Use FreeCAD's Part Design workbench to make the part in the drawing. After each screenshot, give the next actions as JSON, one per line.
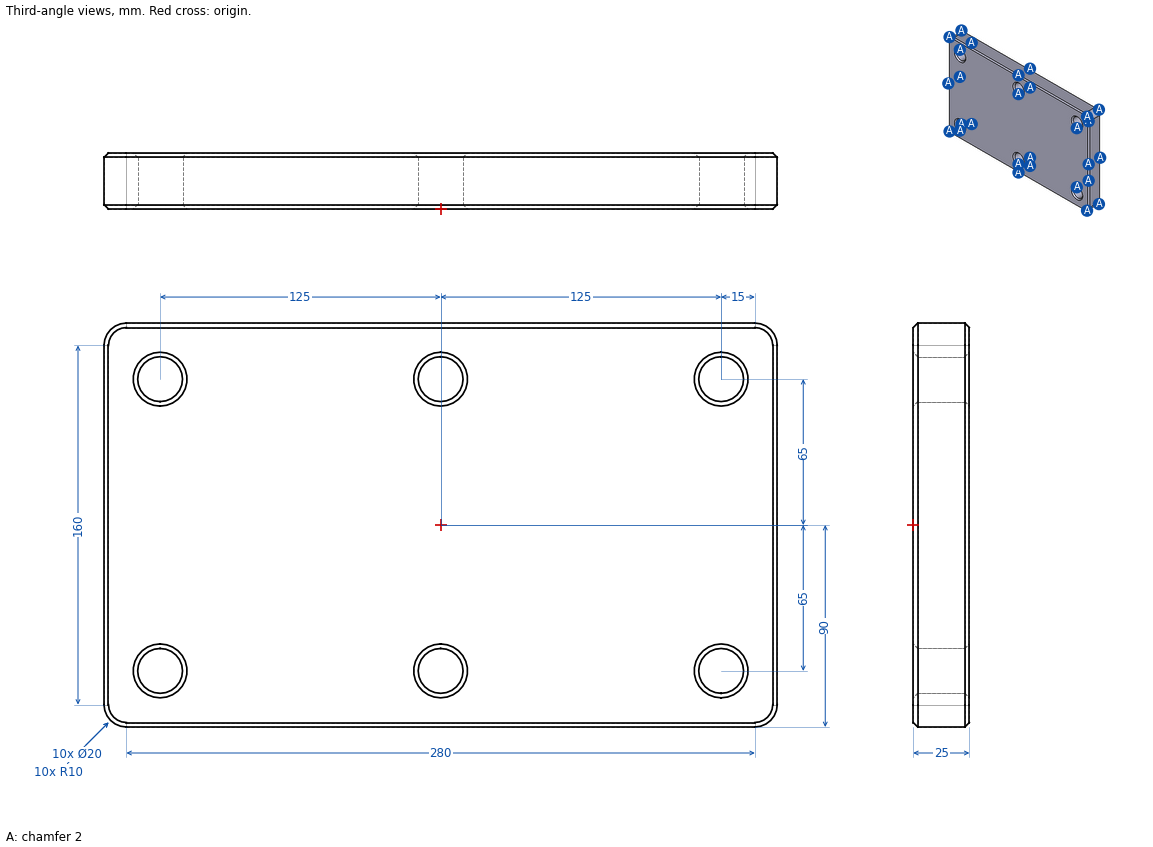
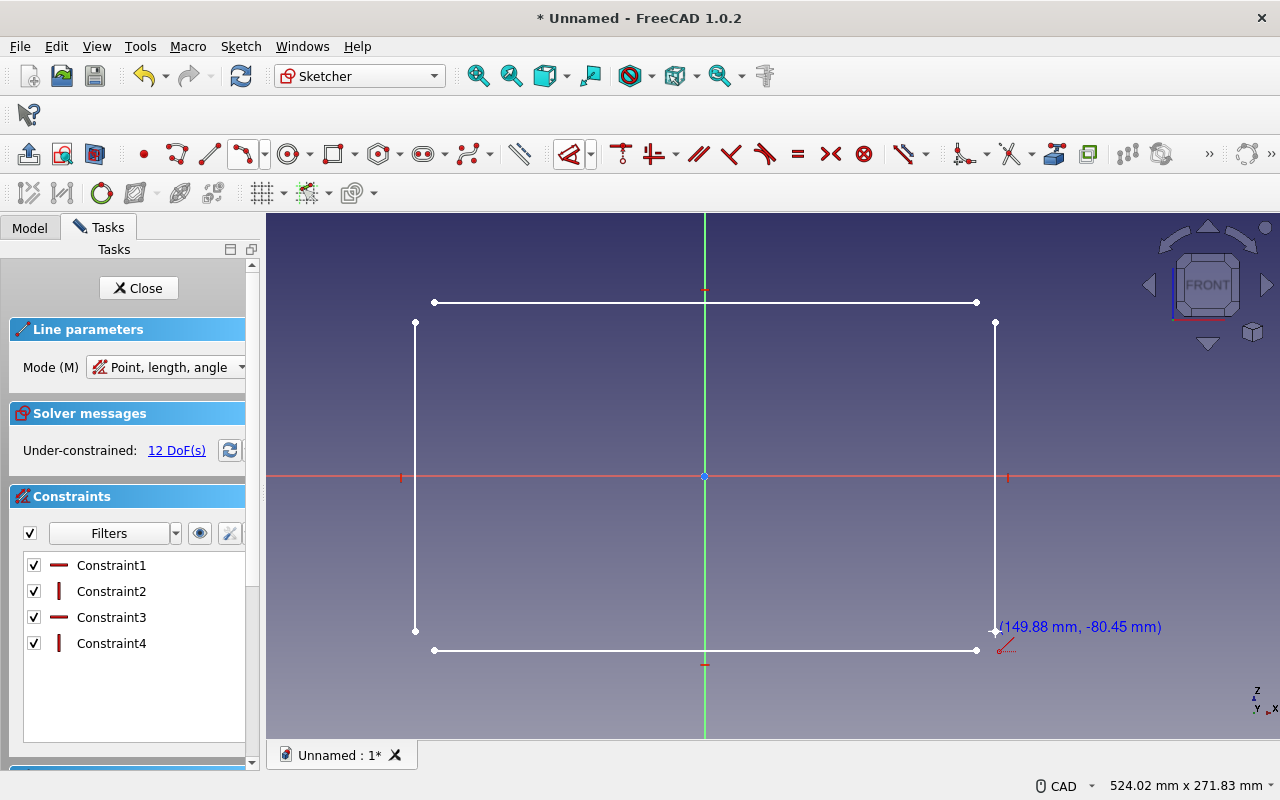
{"action": "left_click", "coordinate": [242, 154]}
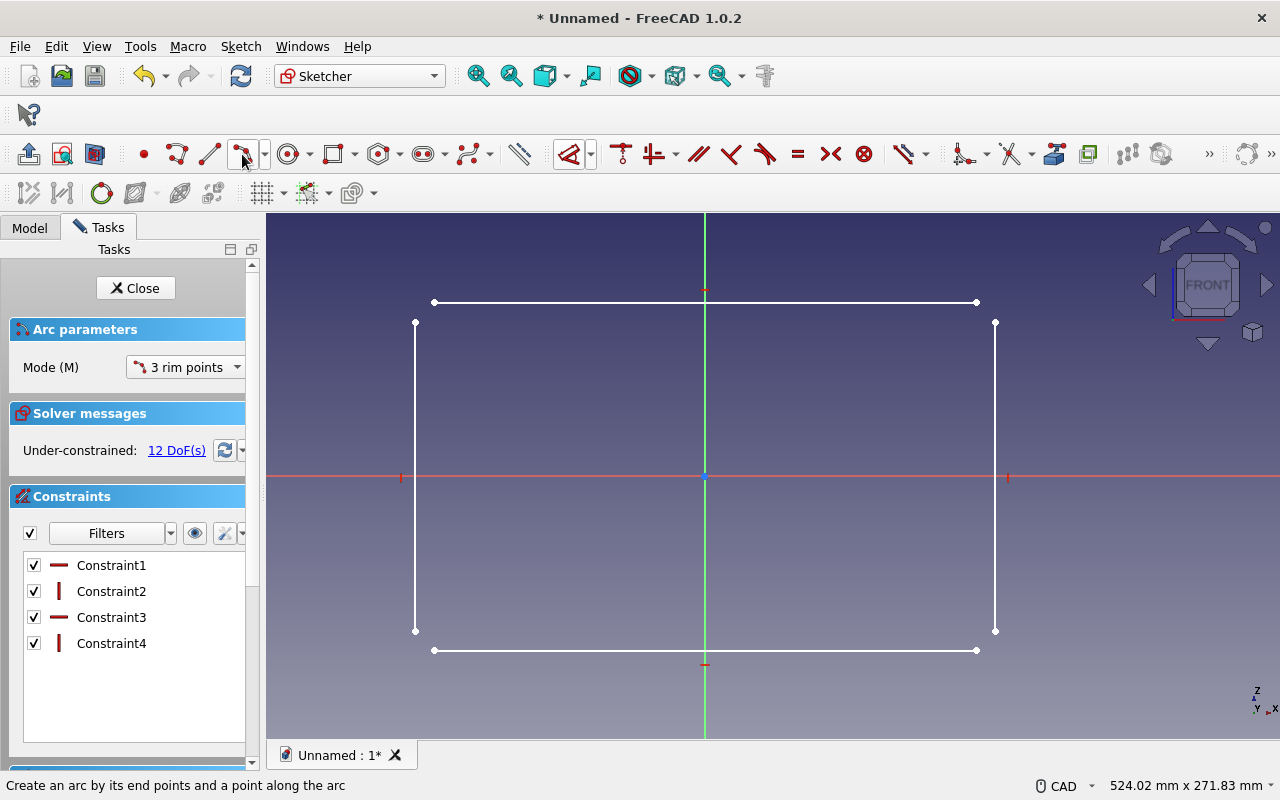
{"action": "left_click", "coordinate": [434, 651]}
{"action": "left_click", "coordinate": [415, 632]}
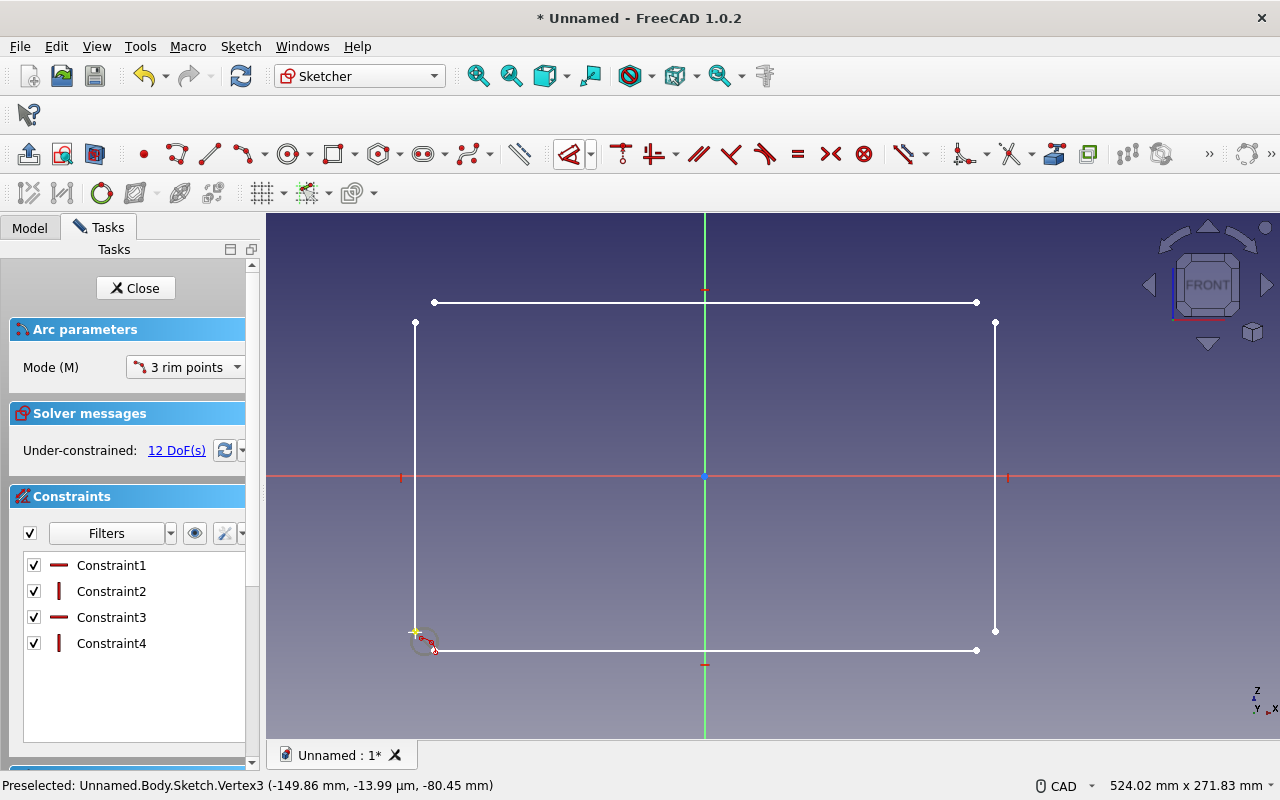
{"action": "scroll", "coordinate": [420, 645], "scroll_direction": "up", "scroll_amount": 6}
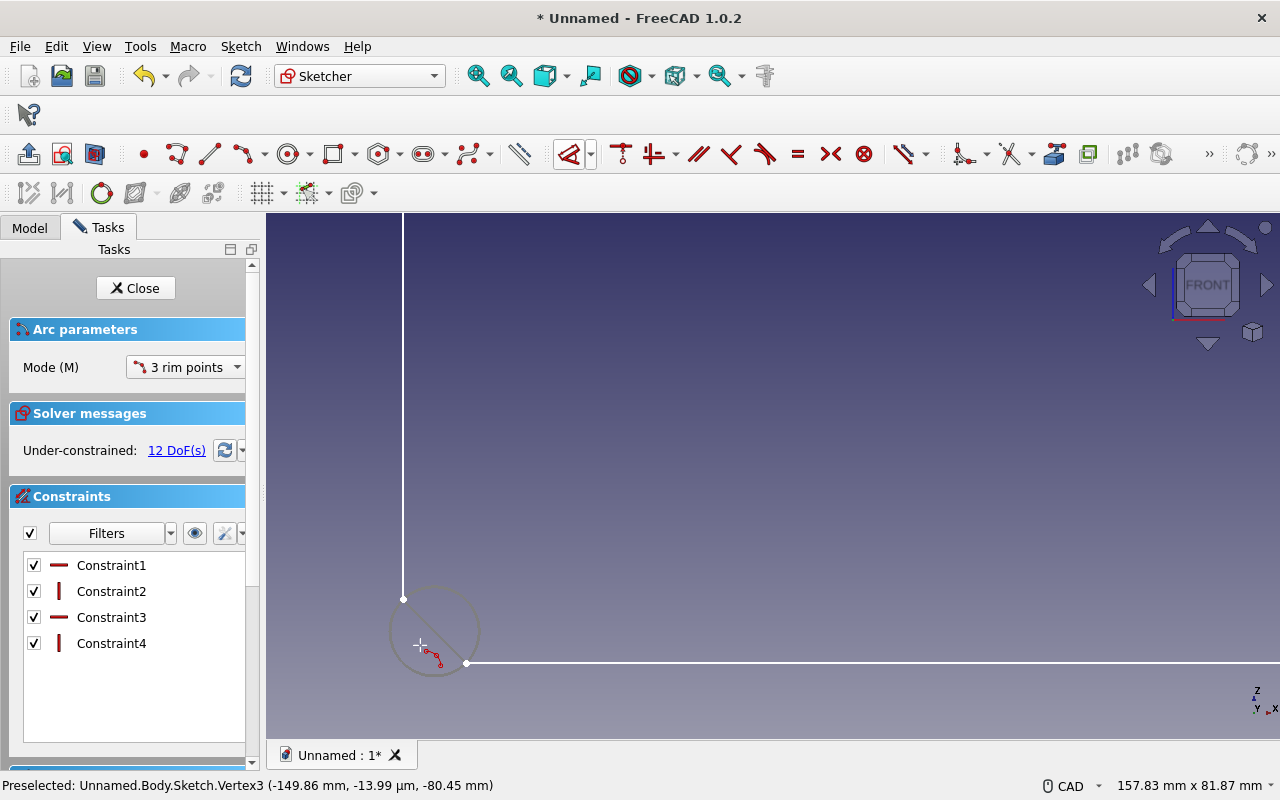
{"action": "left_click", "coordinate": [421, 642]}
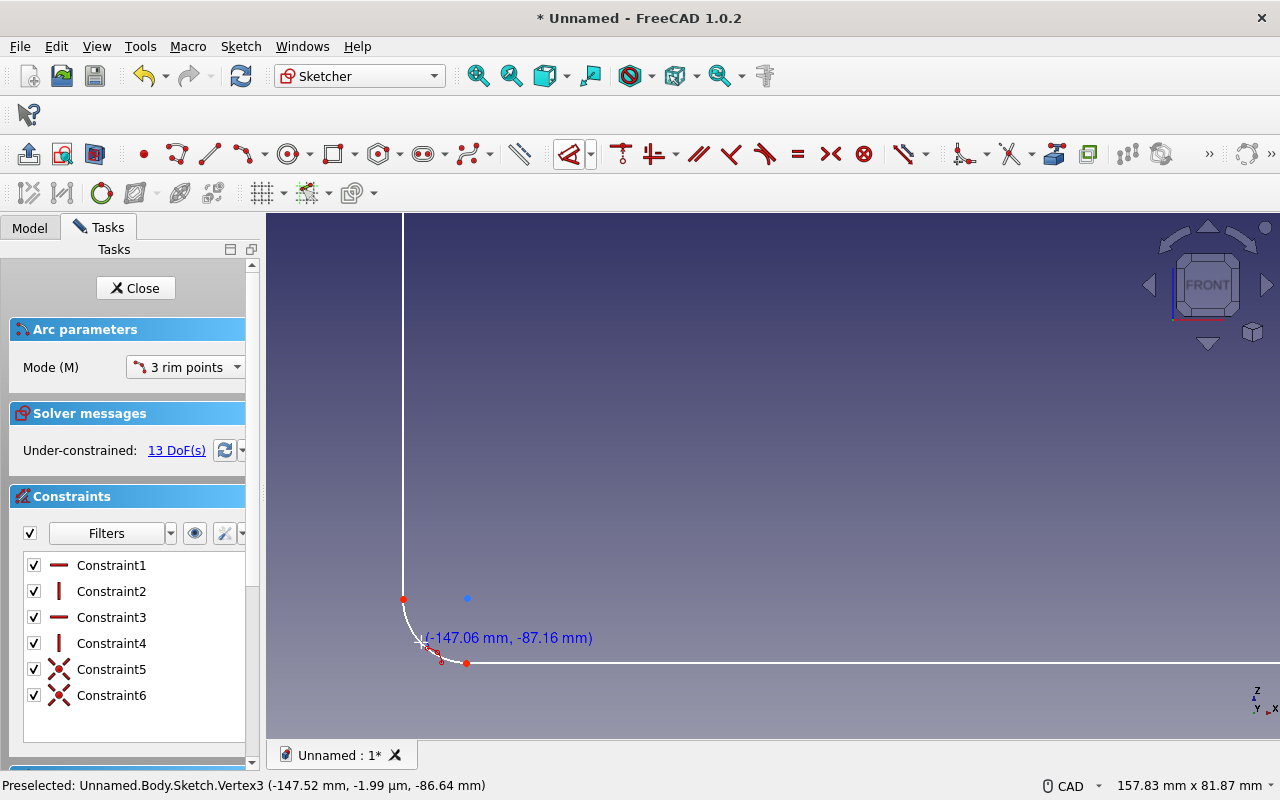
{"action": "scroll", "coordinate": [419, 645], "scroll_direction": "down", "scroll_amount": 6}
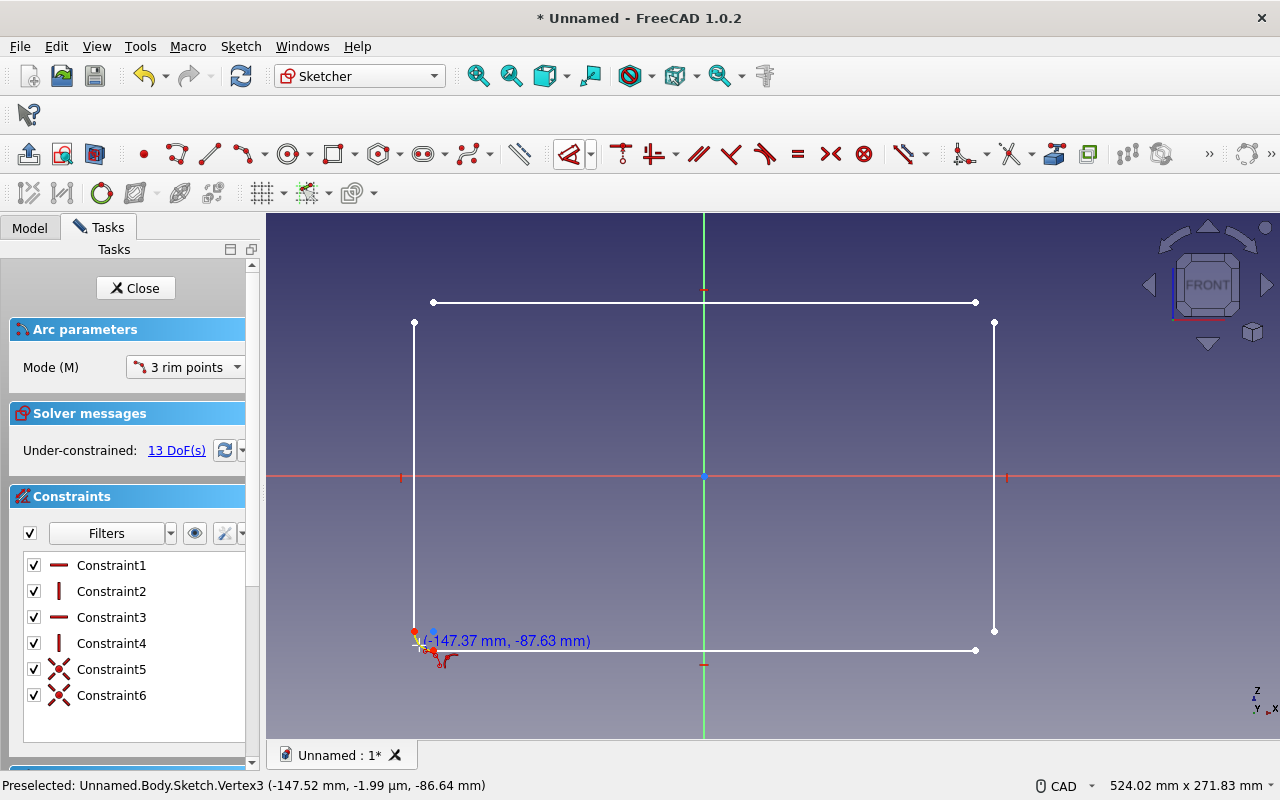
{"action": "left_click", "coordinate": [414, 323]}
{"action": "left_click", "coordinate": [433, 303]}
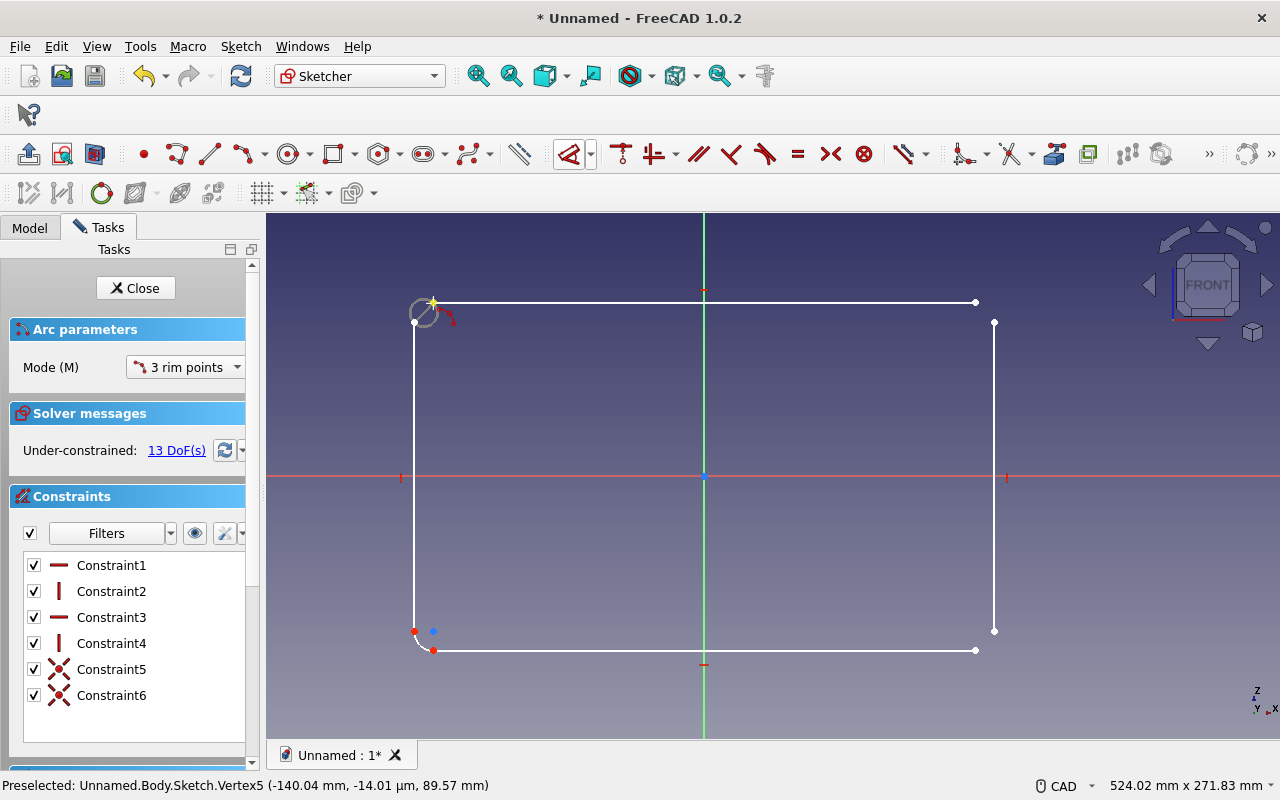
{"action": "scroll", "coordinate": [420, 308], "scroll_direction": "up", "scroll_amount": 6}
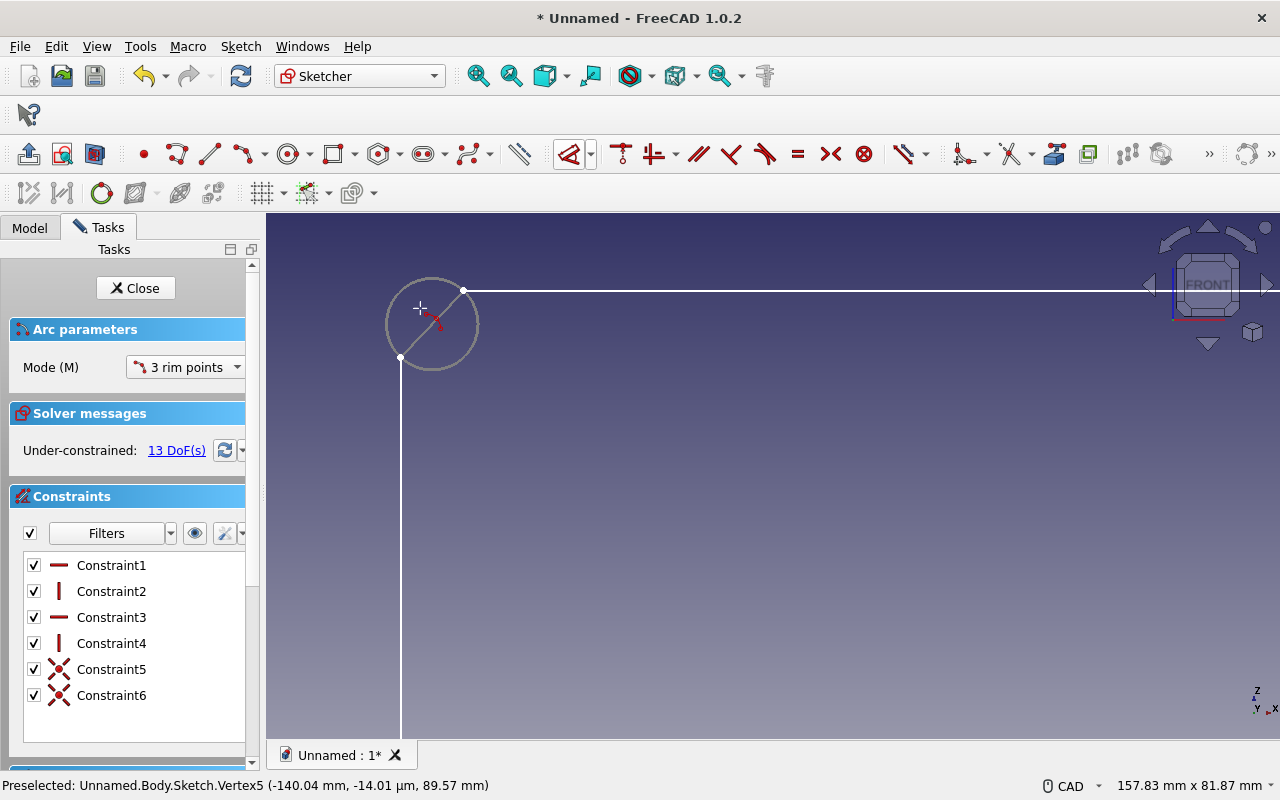
{"action": "left_click", "coordinate": [419, 307]}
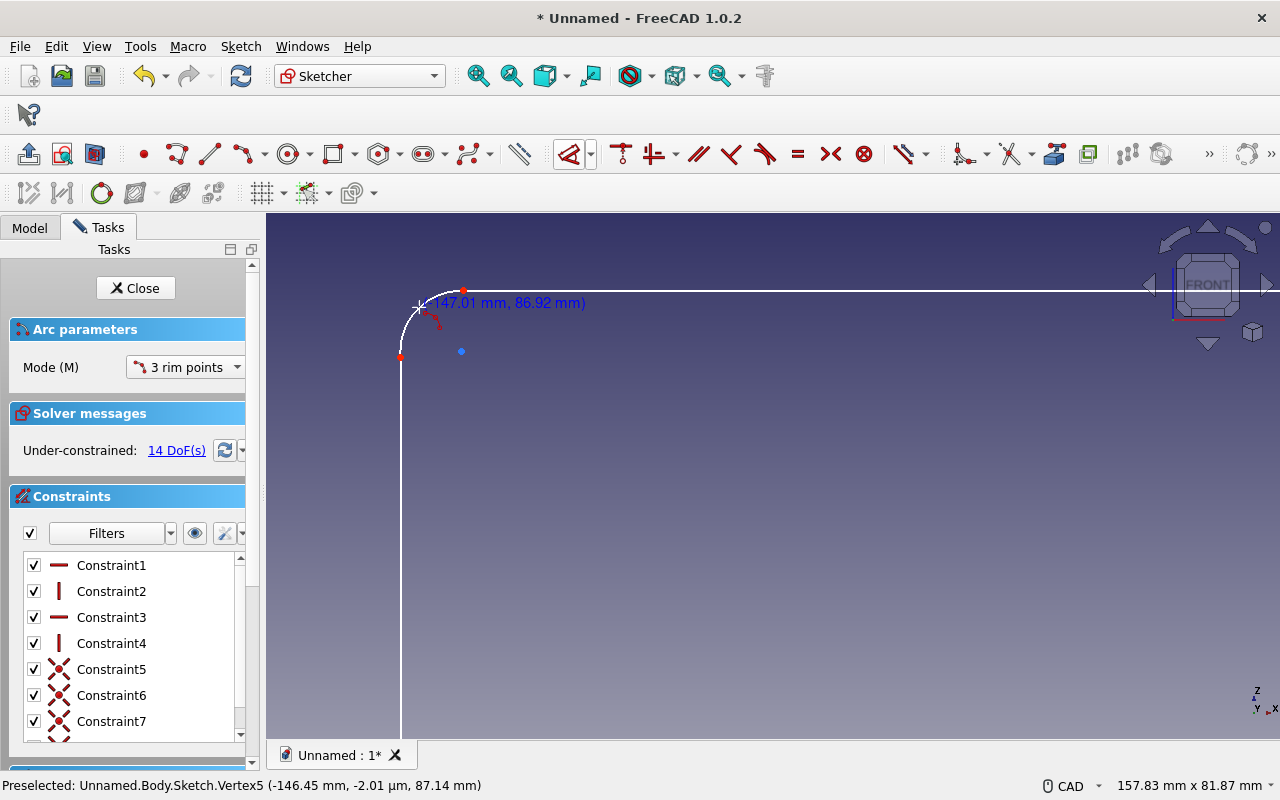
{"action": "scroll", "coordinate": [420, 308], "scroll_direction": "down", "scroll_amount": 6}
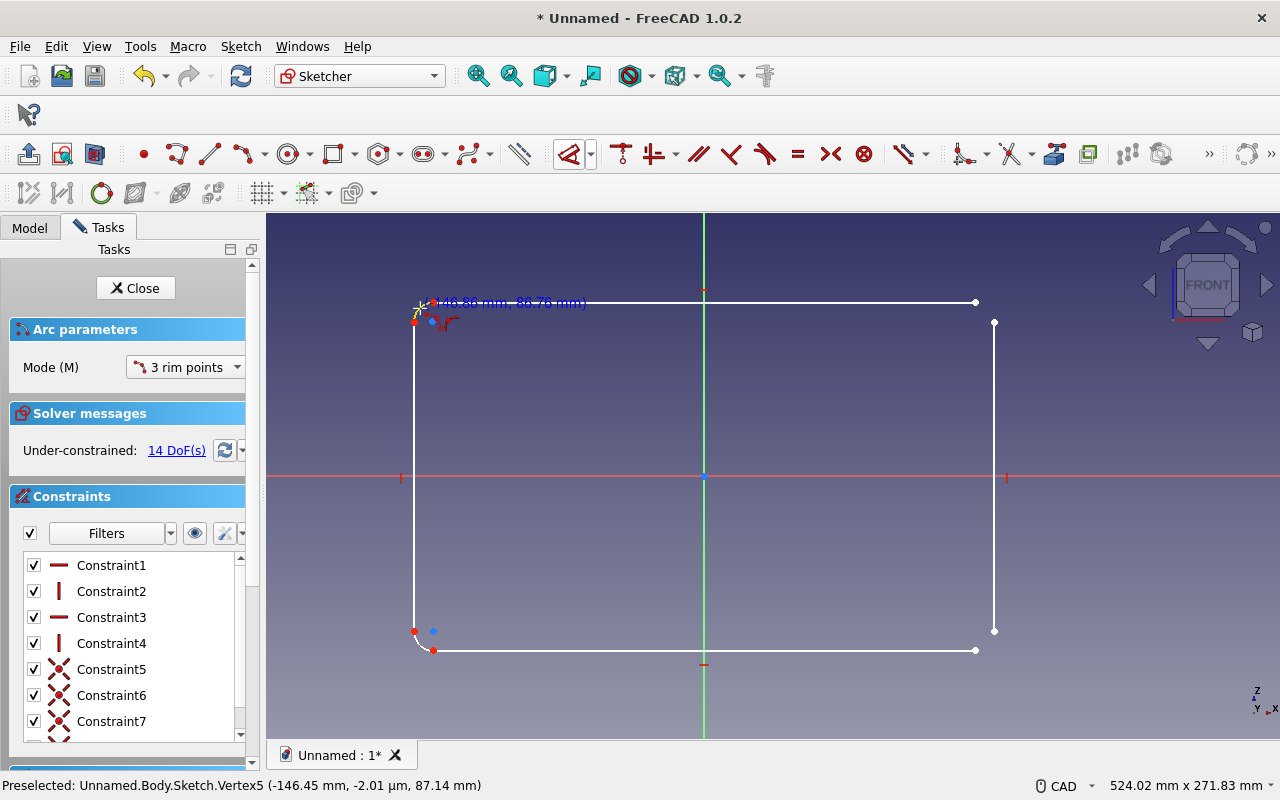
{"action": "left_click", "coordinate": [975, 303]}
{"action": "left_click", "coordinate": [994, 323]}